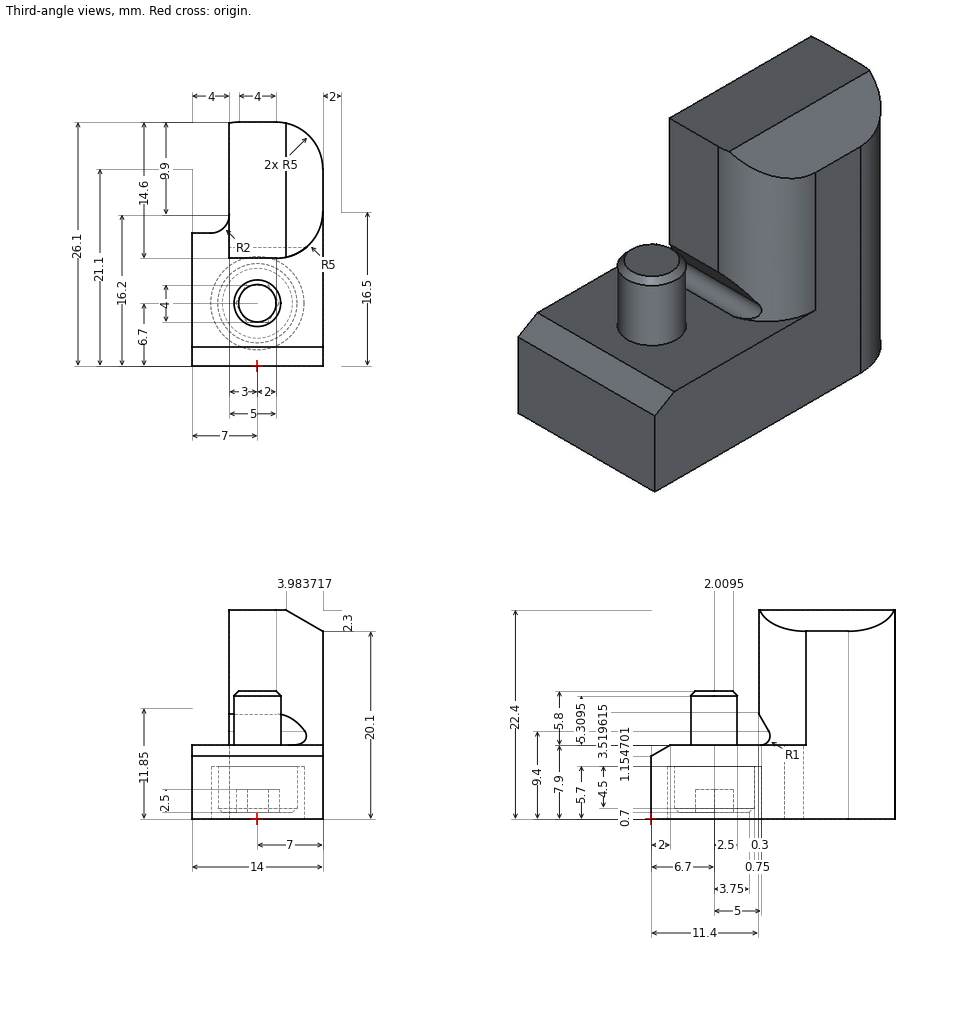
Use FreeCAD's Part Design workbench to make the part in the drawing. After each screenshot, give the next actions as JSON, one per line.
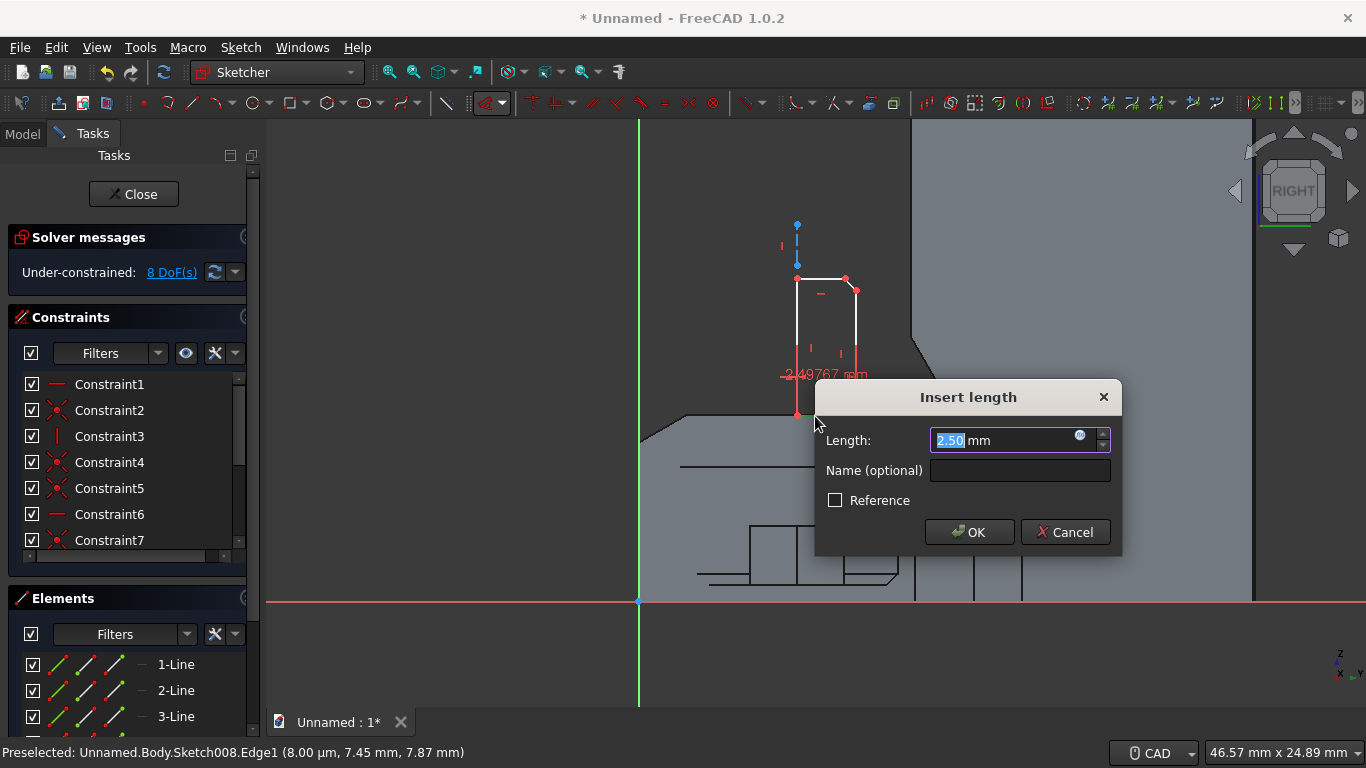
{"action": "type", "text": "2.5"}
{"action": "key", "text": "Return"}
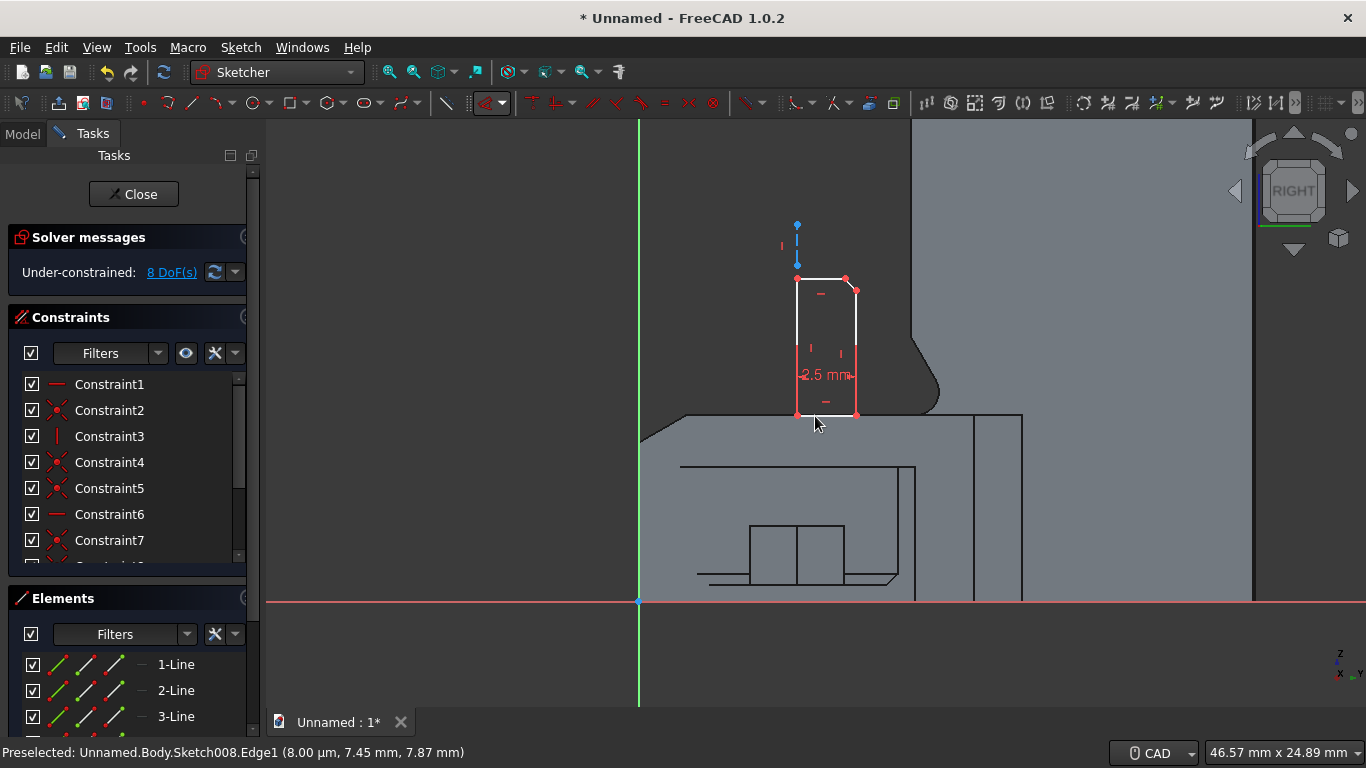
{"action": "left_click", "coordinate": [797, 320]}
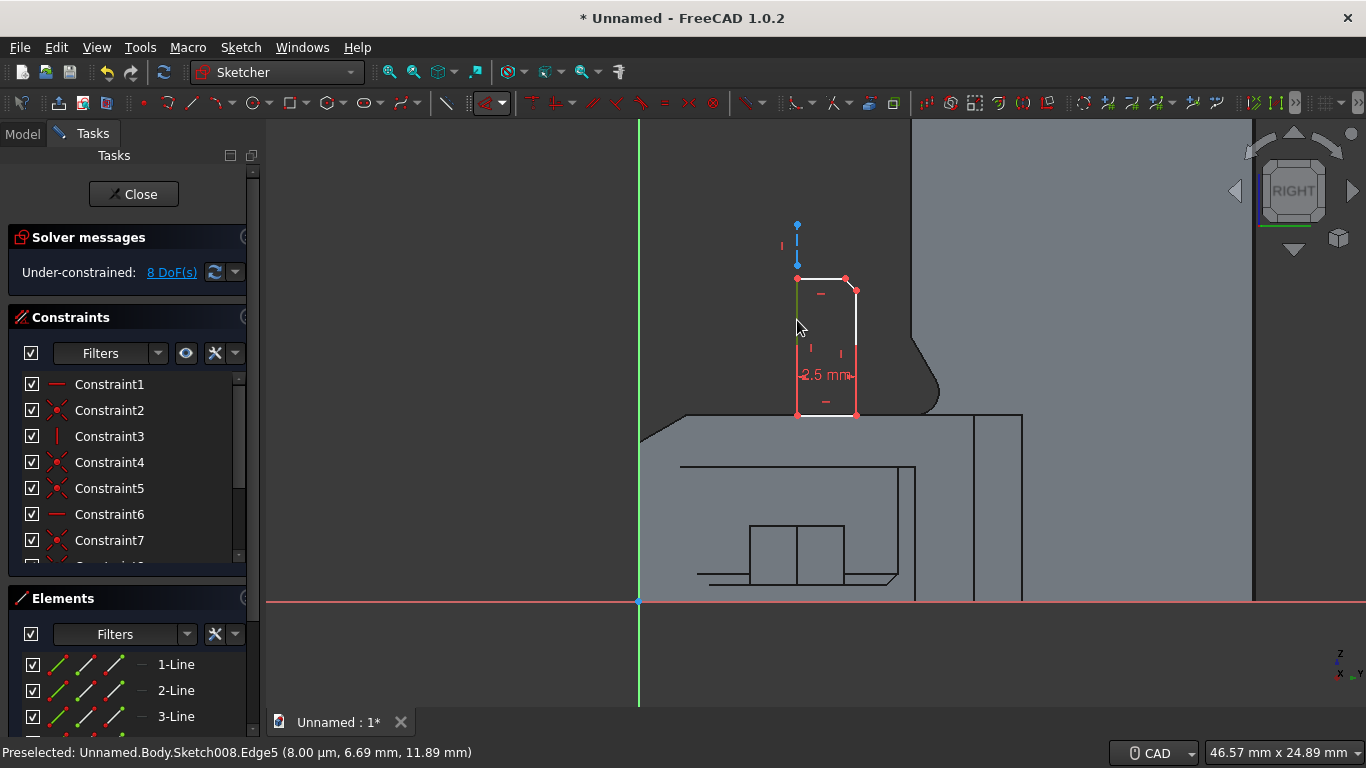
{"action": "left_click", "coordinate": [504, 104]}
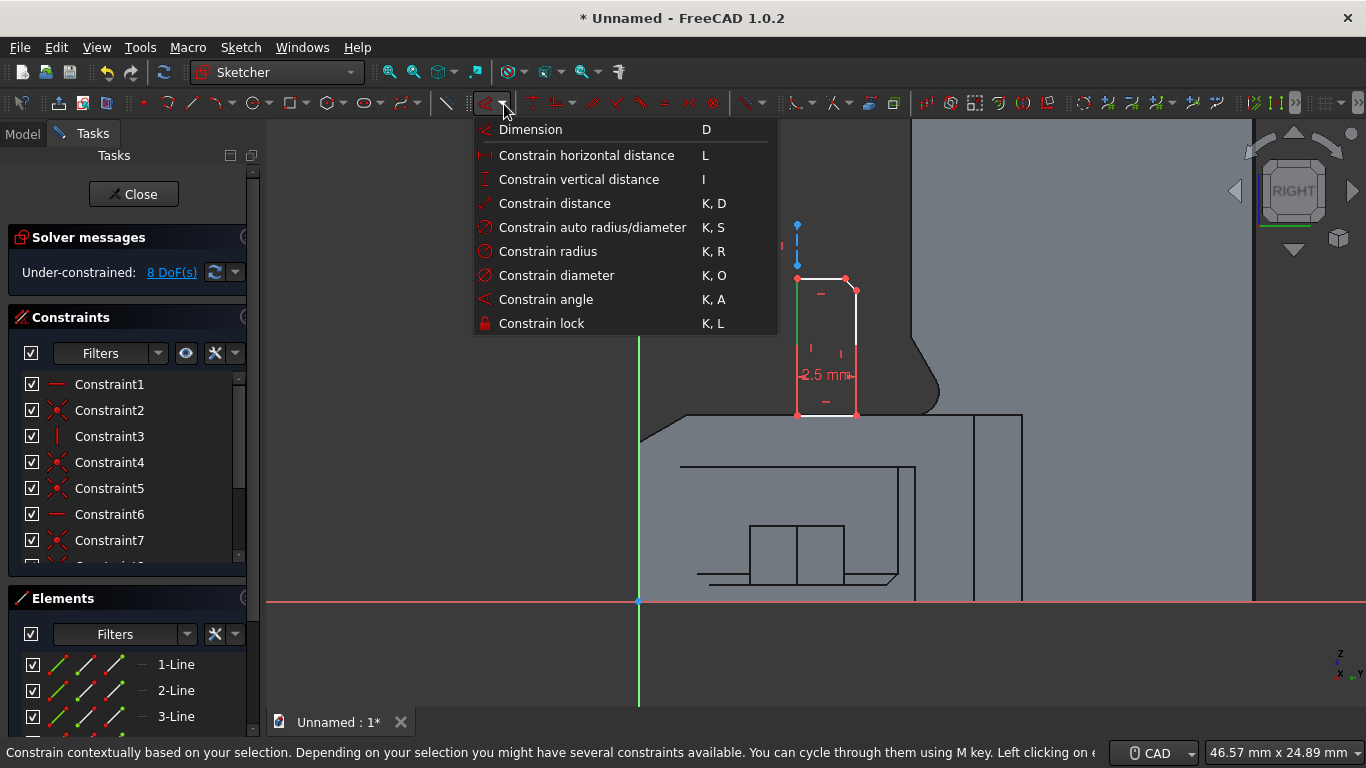
{"action": "left_click", "coordinate": [626, 179]}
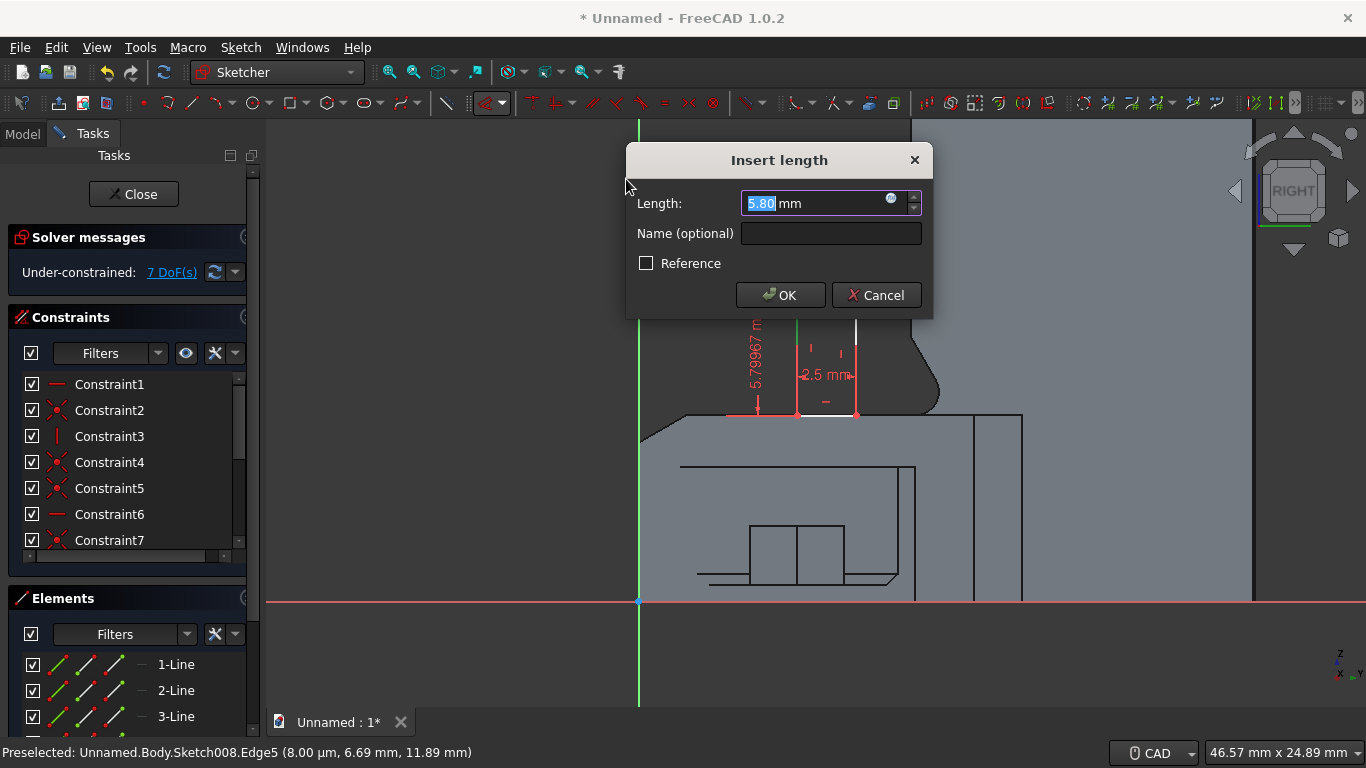
{"action": "type", "text": "5.8"}
{"action": "key", "text": "Return"}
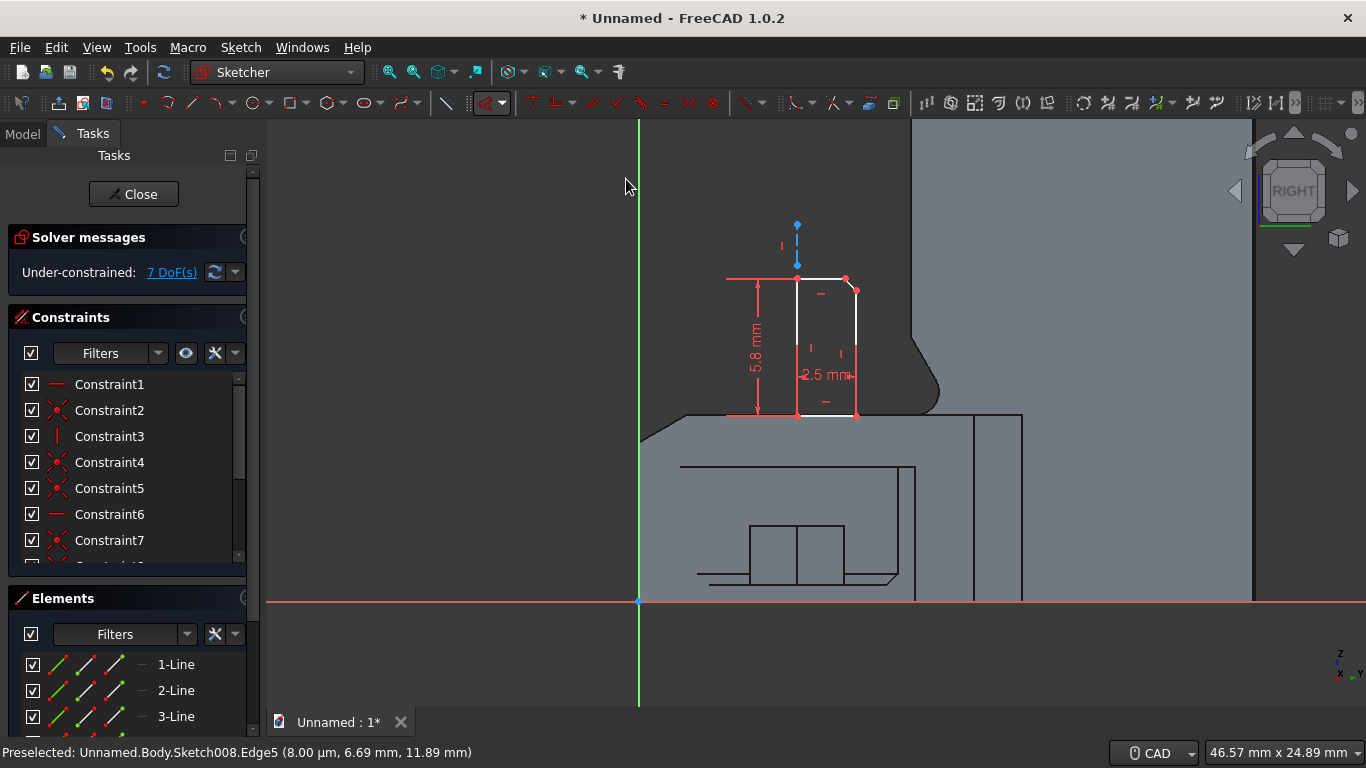
{"action": "left_click", "coordinate": [797, 416]}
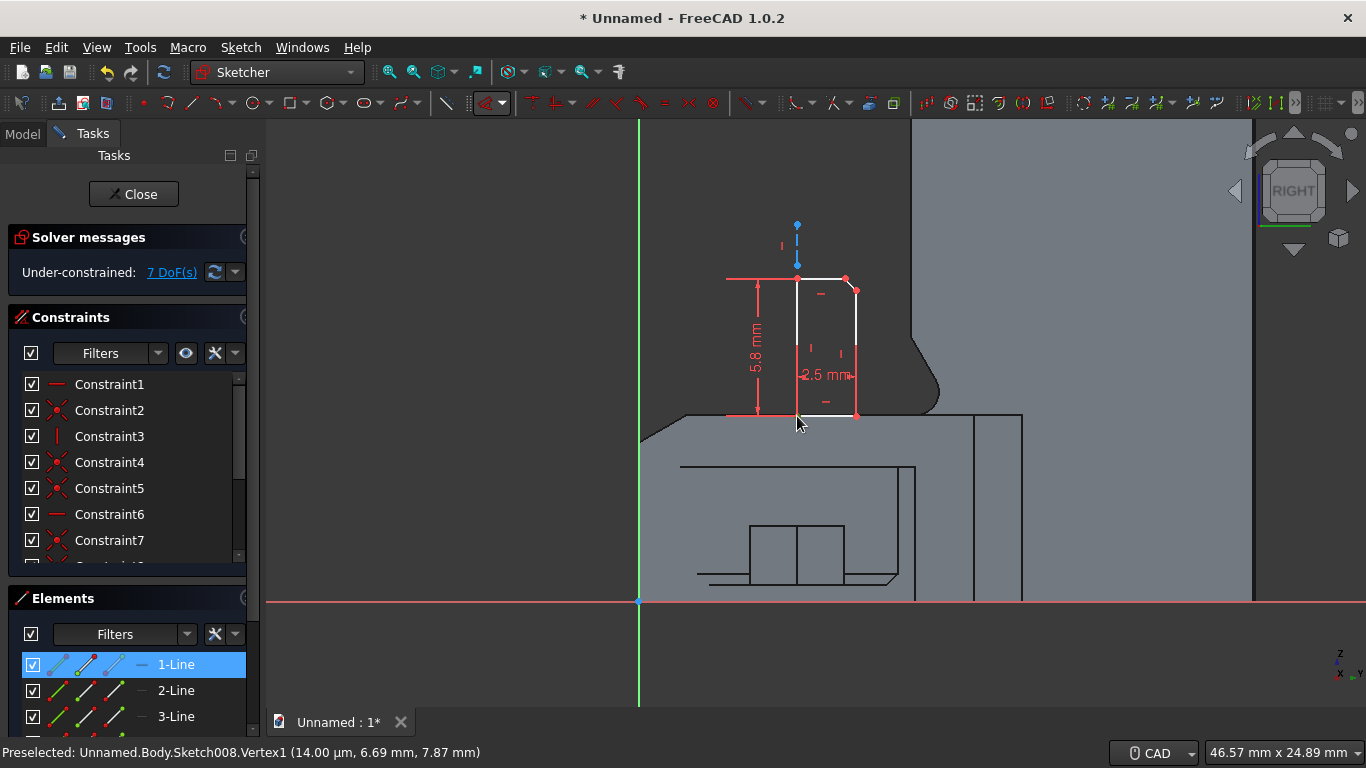
{"action": "left_click", "coordinate": [504, 104]}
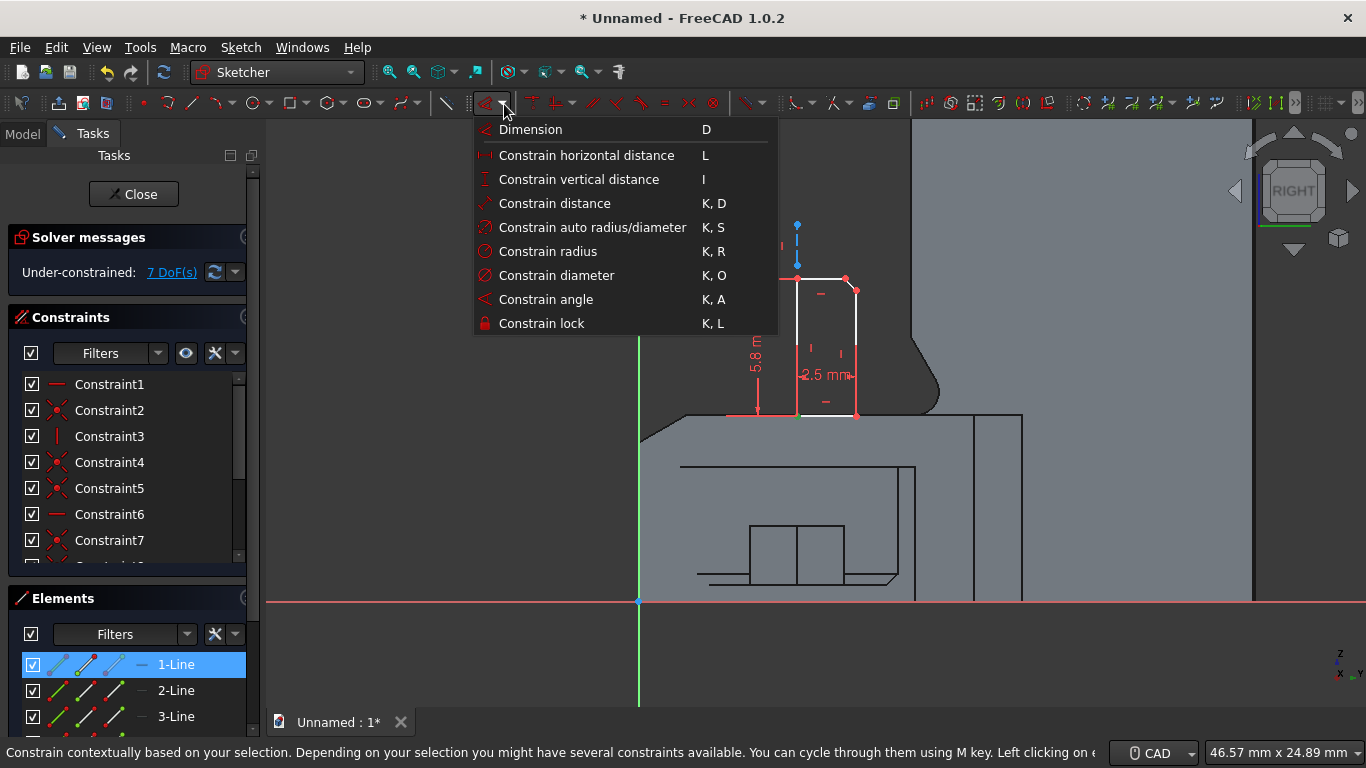
{"action": "left_click", "coordinate": [626, 155]}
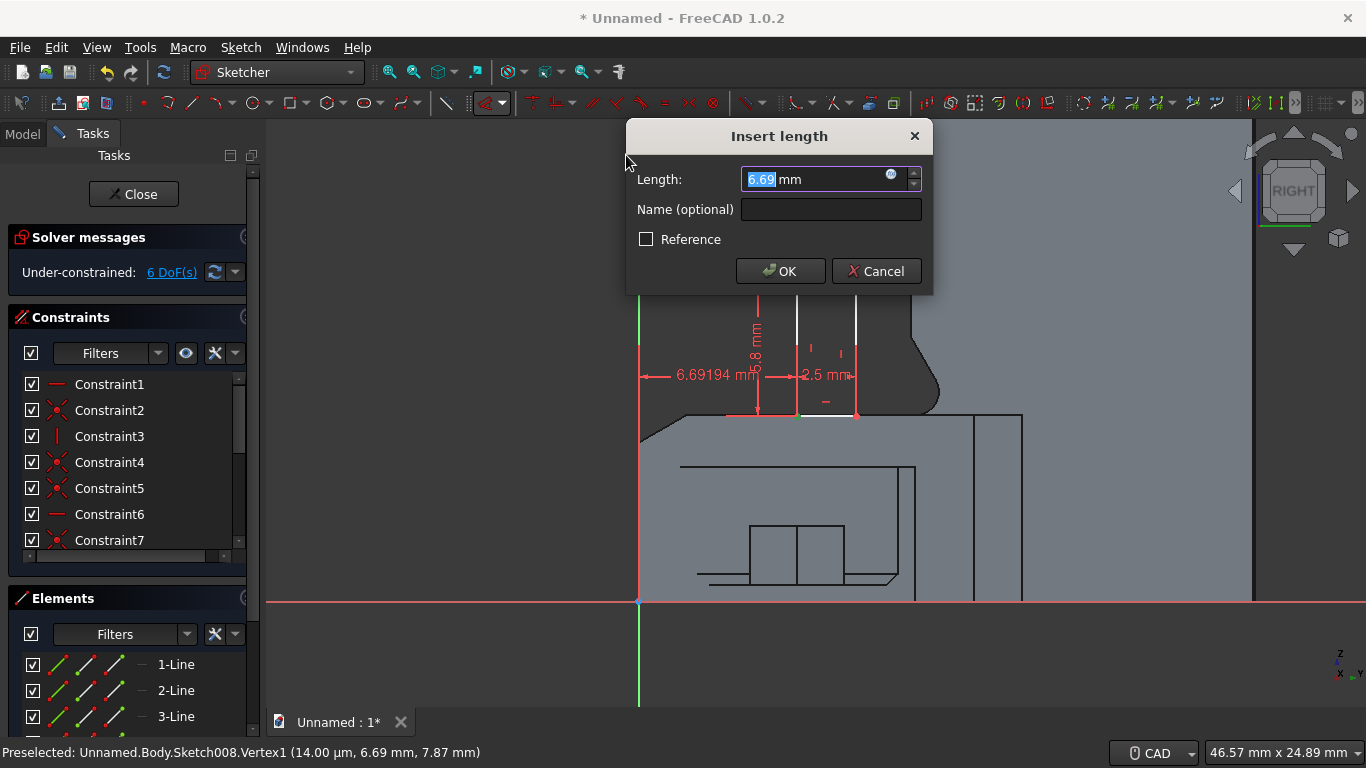
{"action": "type", "text": "6.7"}
{"action": "key", "text": "Return"}